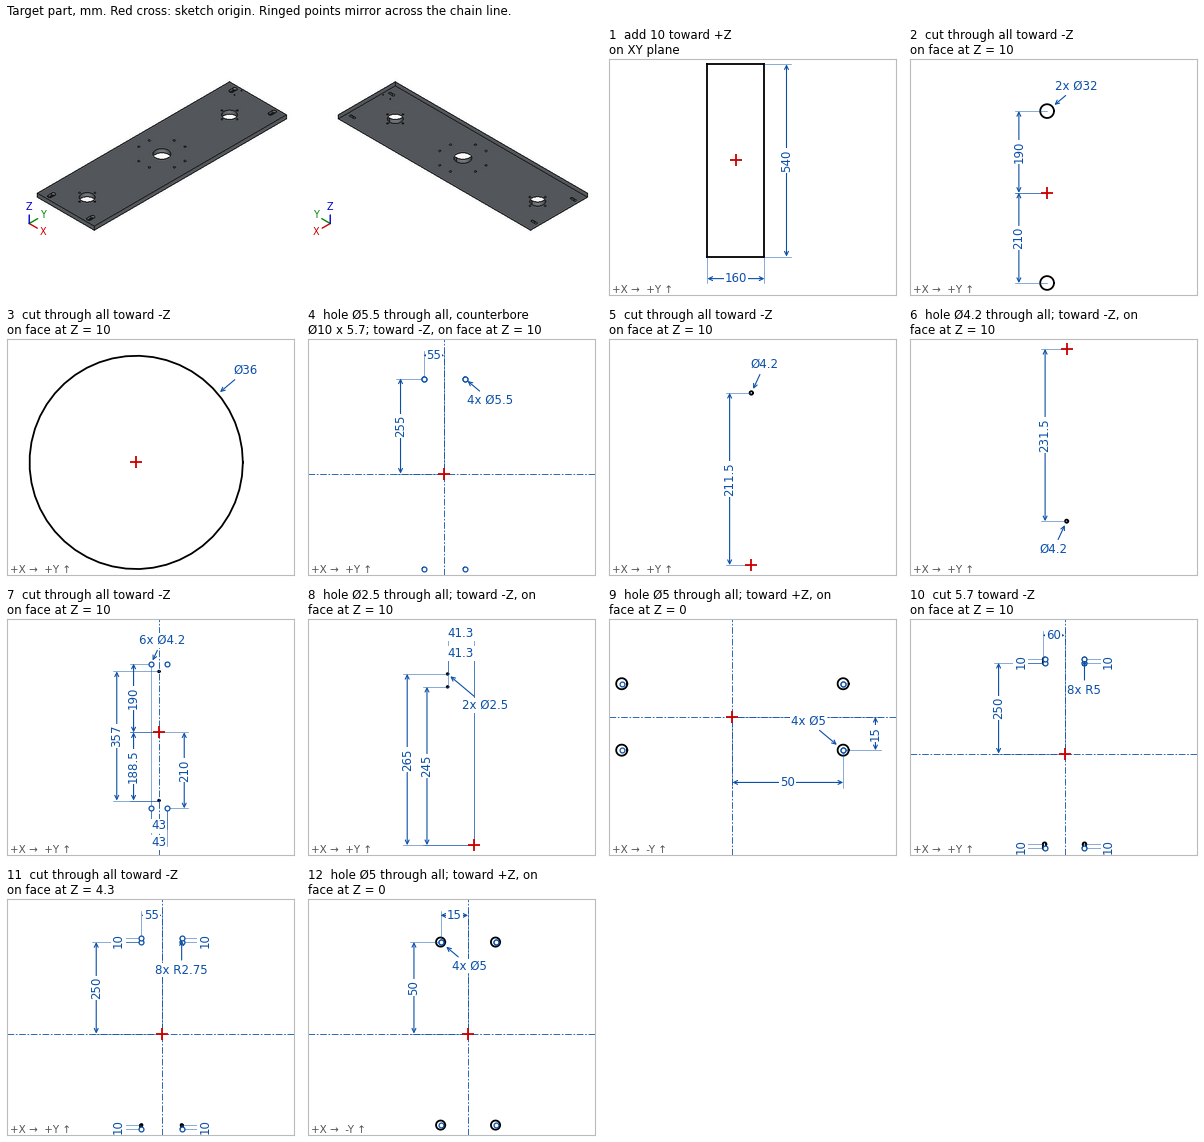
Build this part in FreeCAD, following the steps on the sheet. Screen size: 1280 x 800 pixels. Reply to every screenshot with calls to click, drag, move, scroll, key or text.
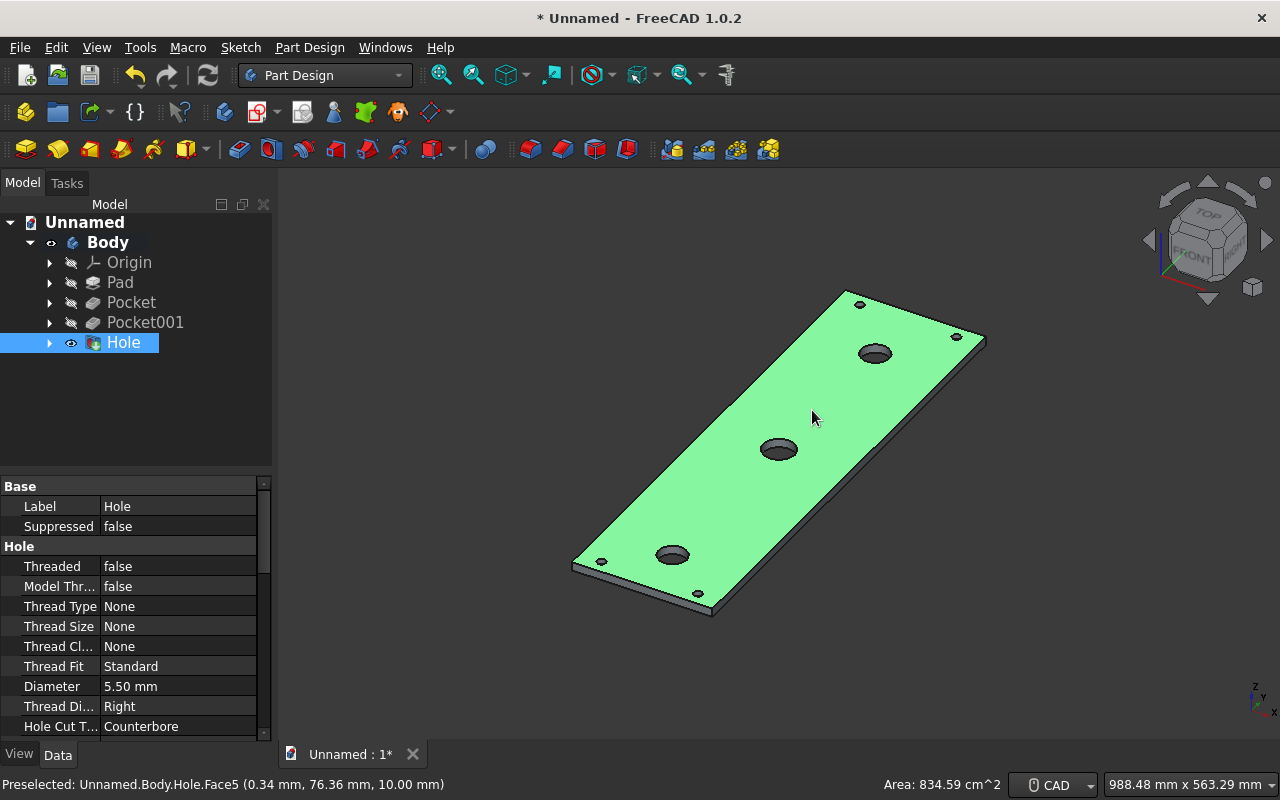
click(258, 112)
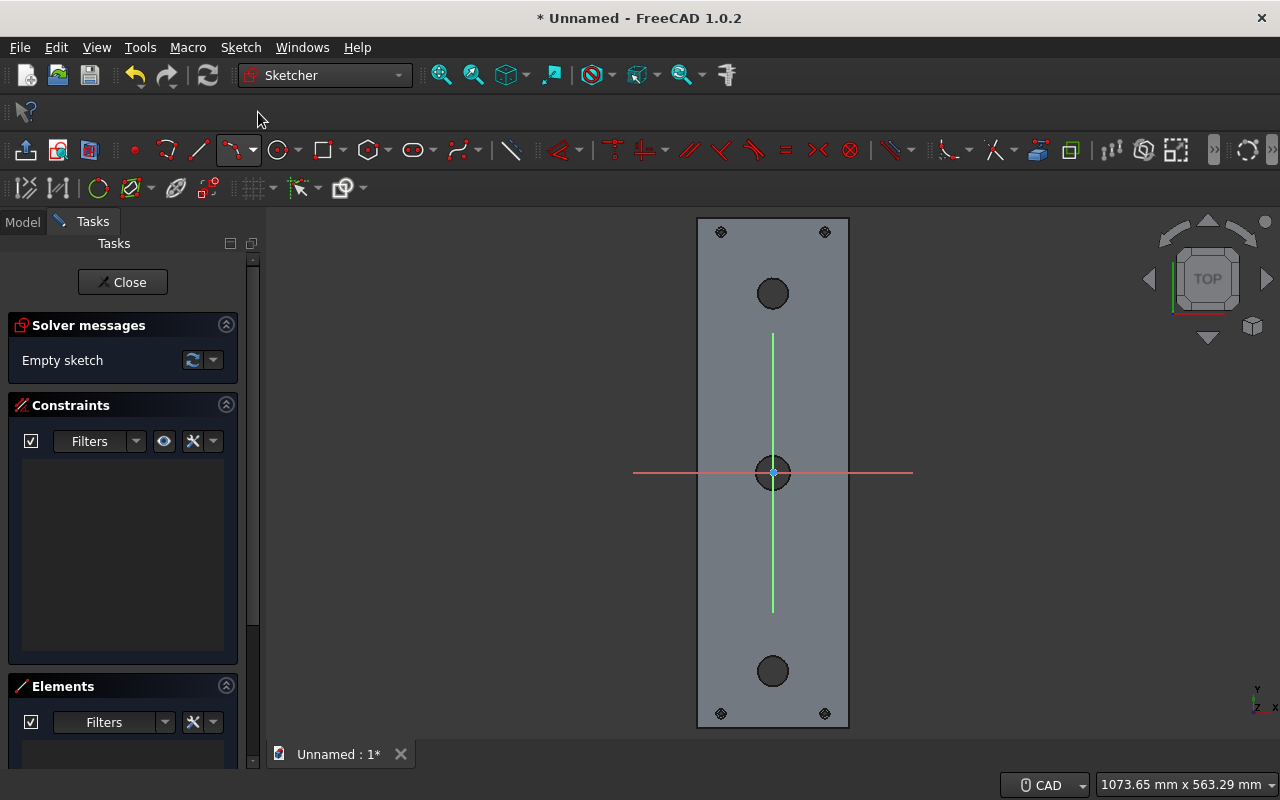
scroll(777, 263, up, 15)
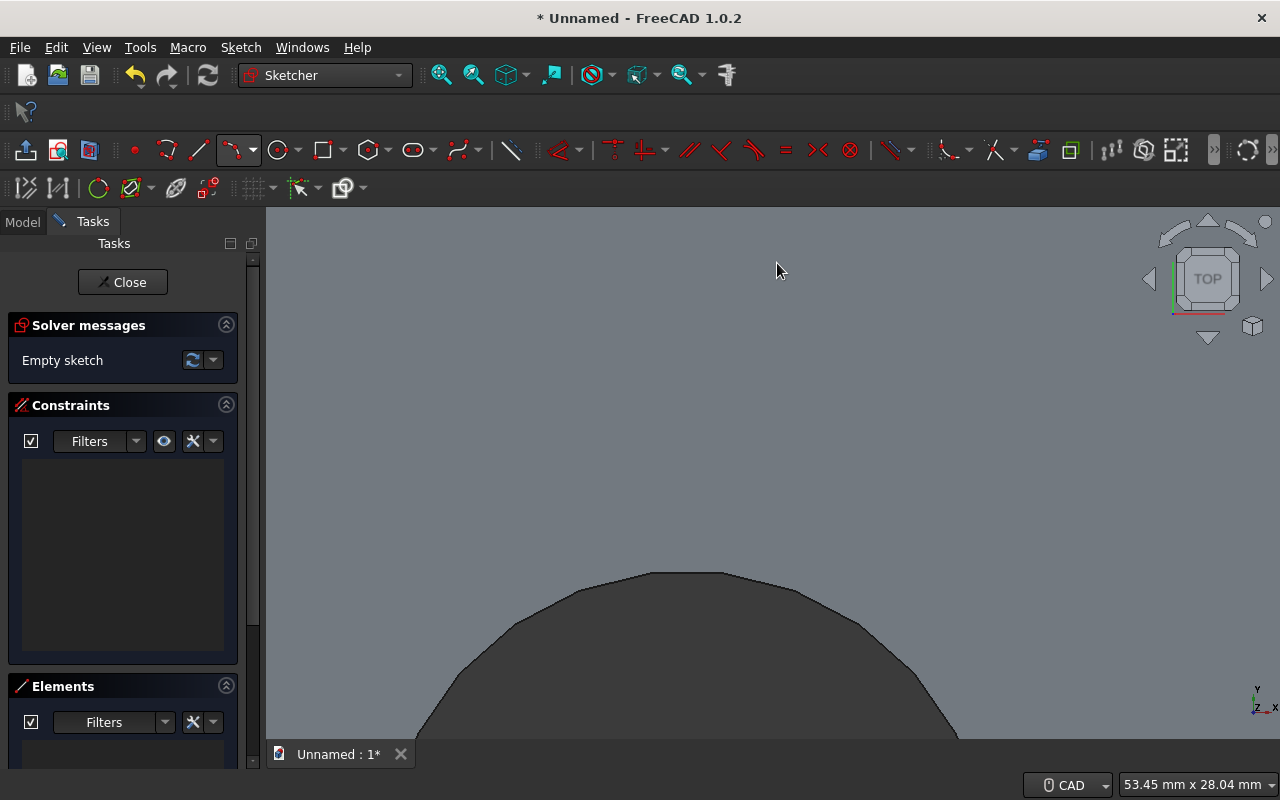
scroll(681, 465, up, 7)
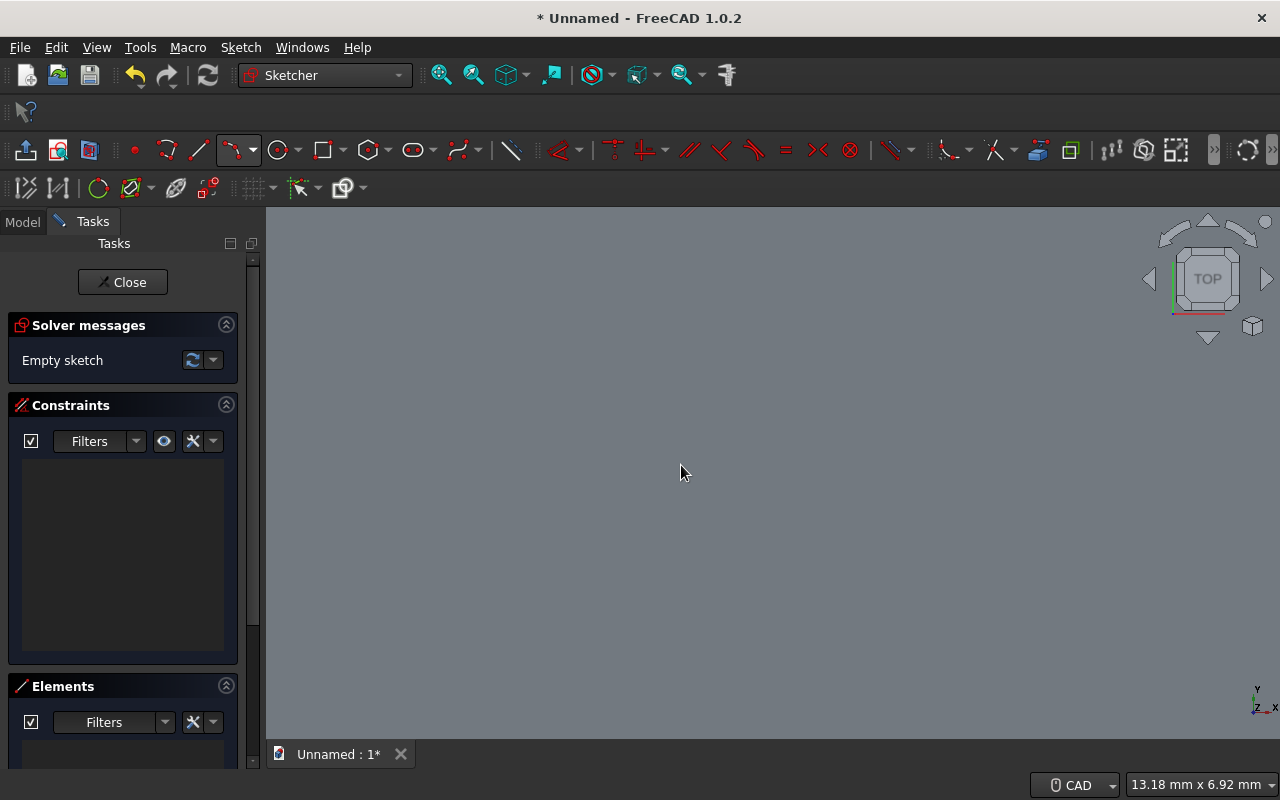
key(g)
key(c)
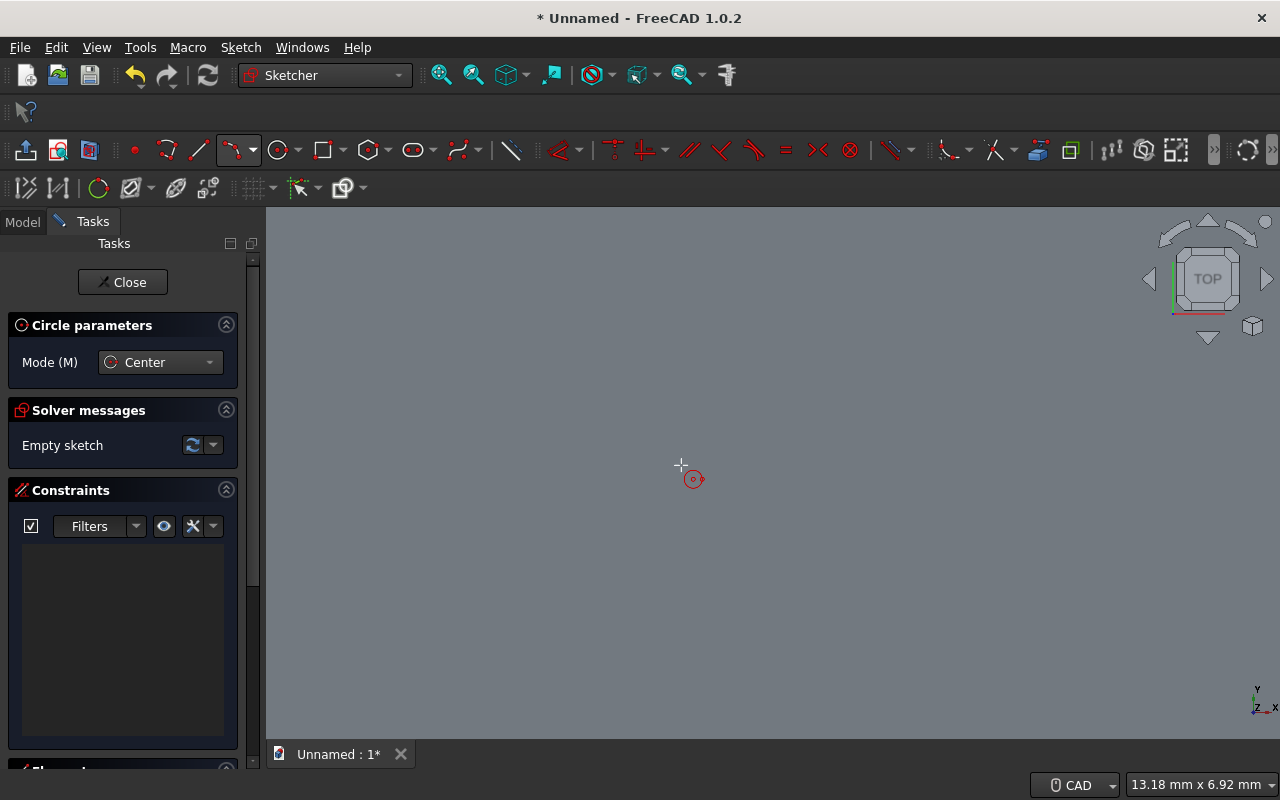
click(704, 471)
move(818, 357)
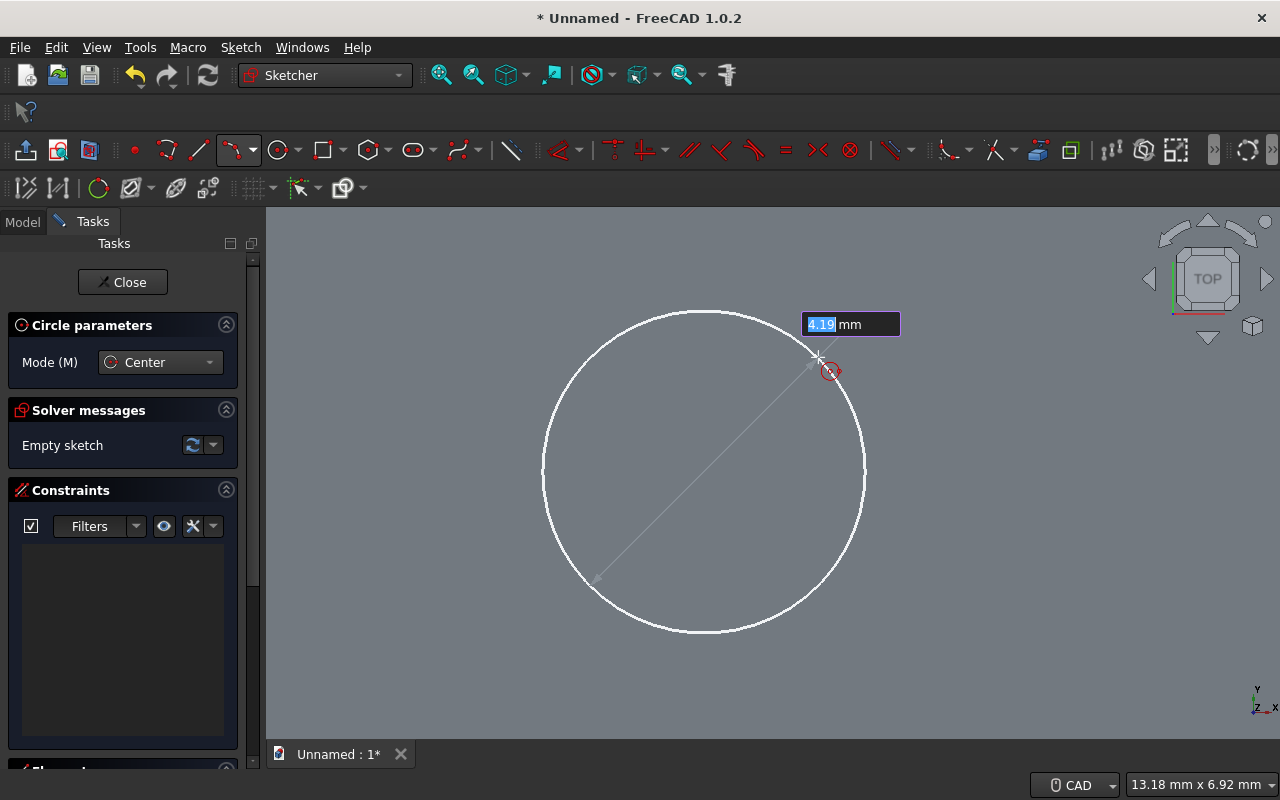
text(4.2)
key(Return)
key(Escape)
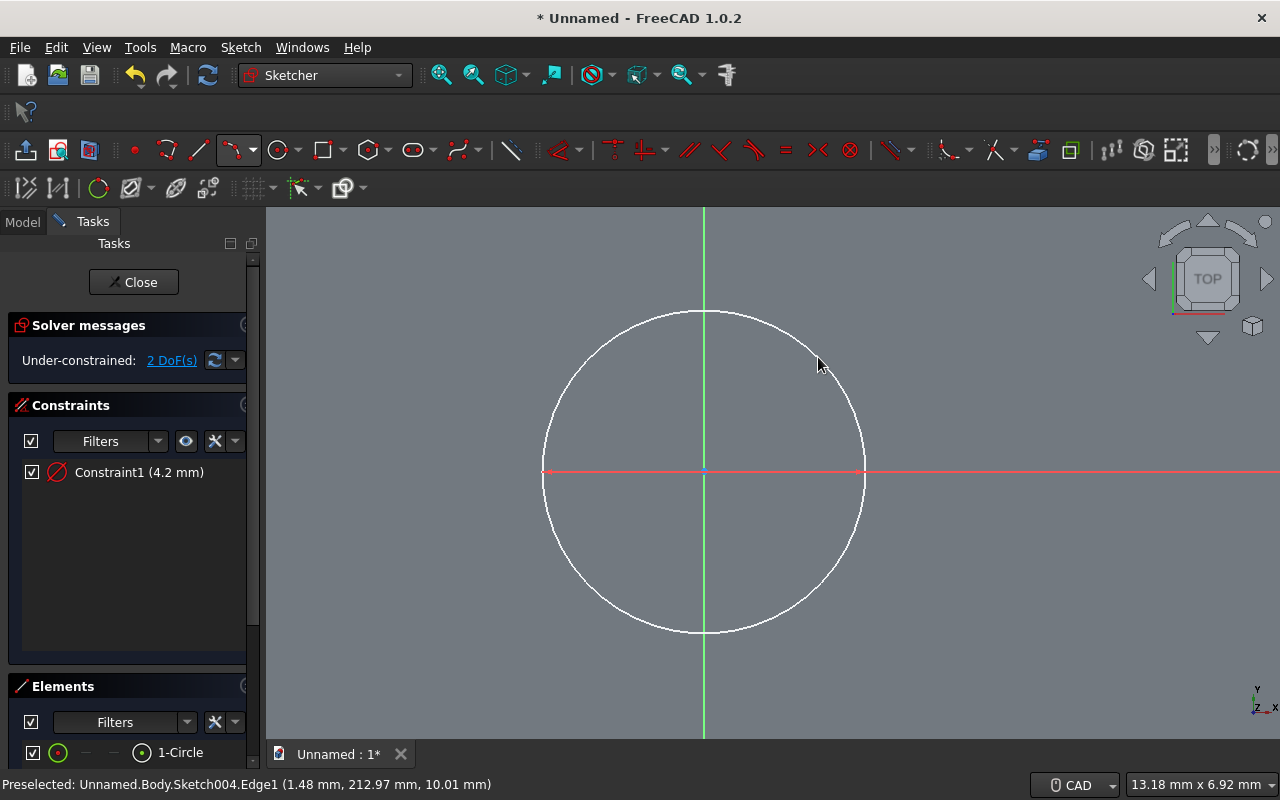
click(704, 472)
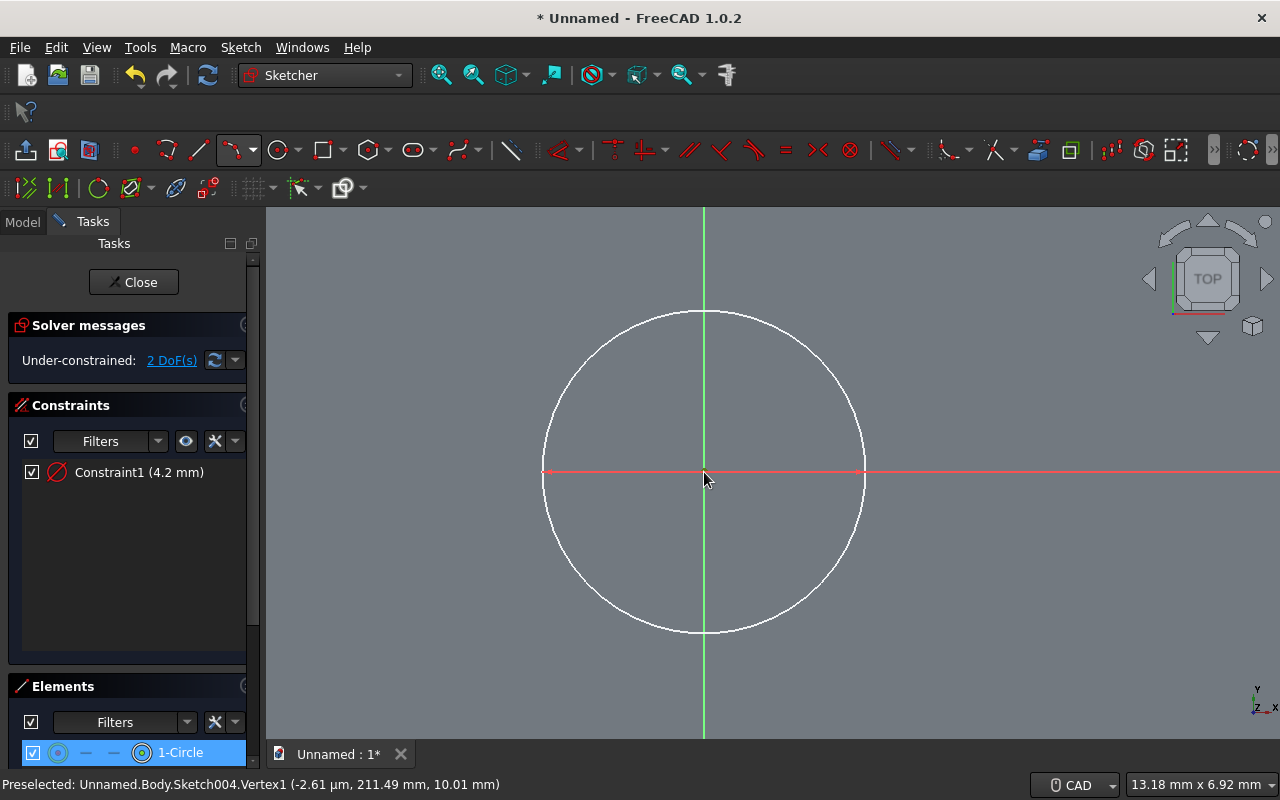
click(704, 677)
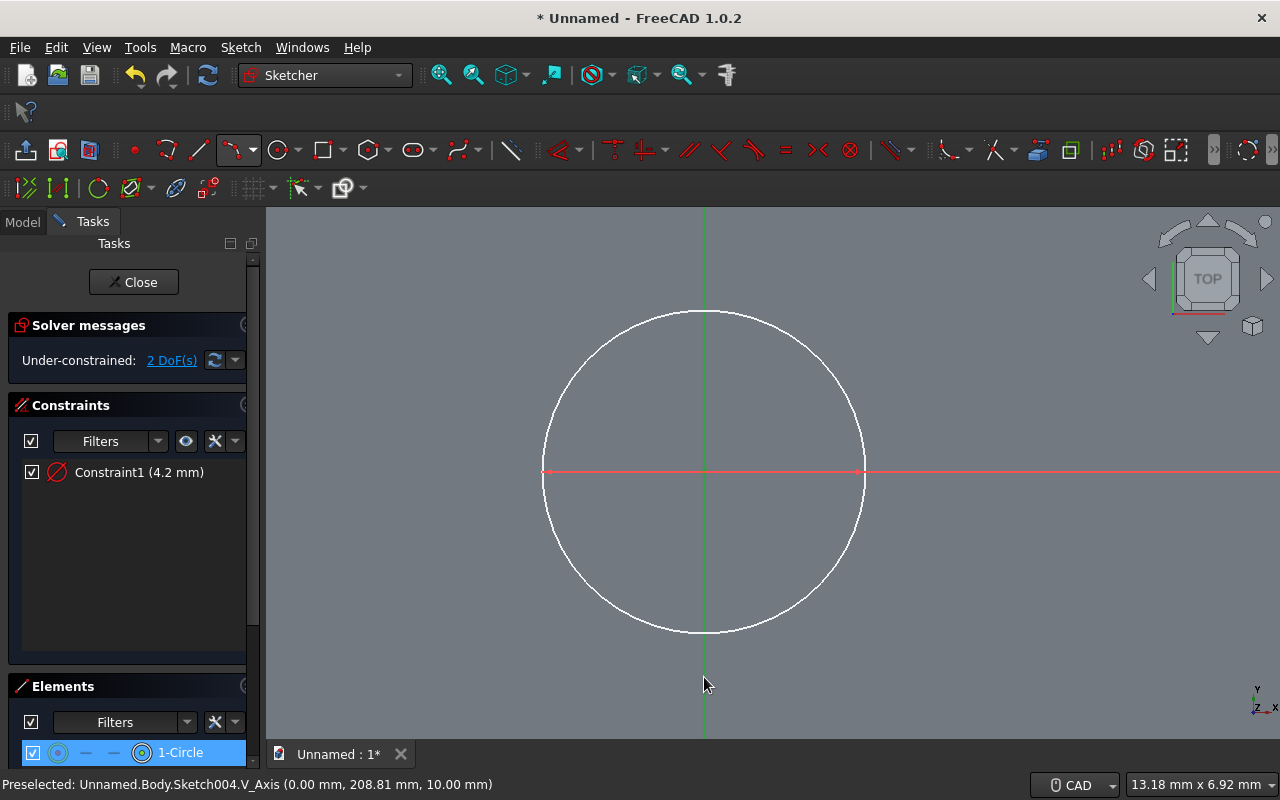
click(614, 150)